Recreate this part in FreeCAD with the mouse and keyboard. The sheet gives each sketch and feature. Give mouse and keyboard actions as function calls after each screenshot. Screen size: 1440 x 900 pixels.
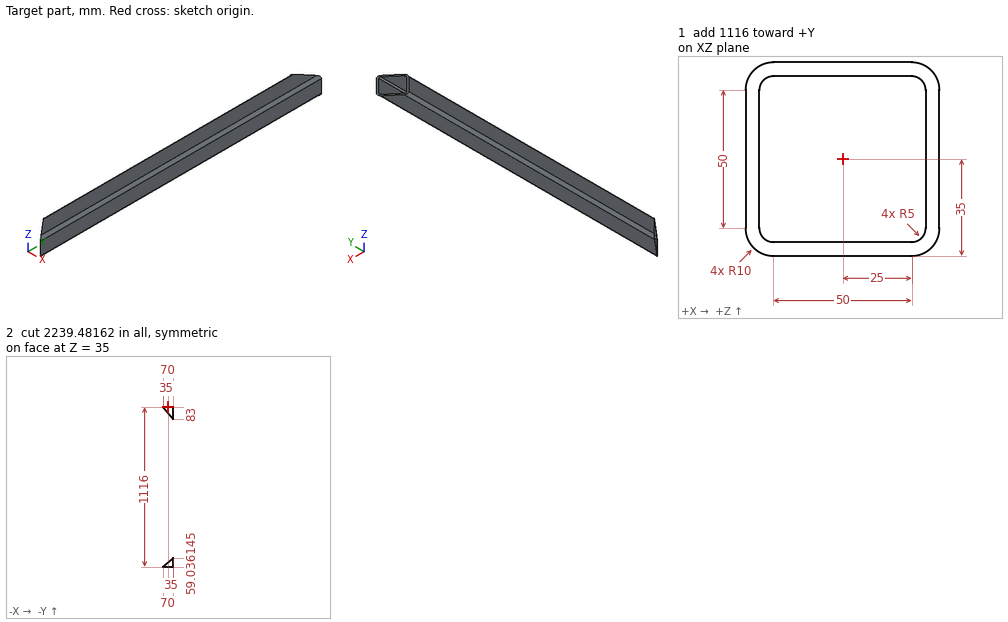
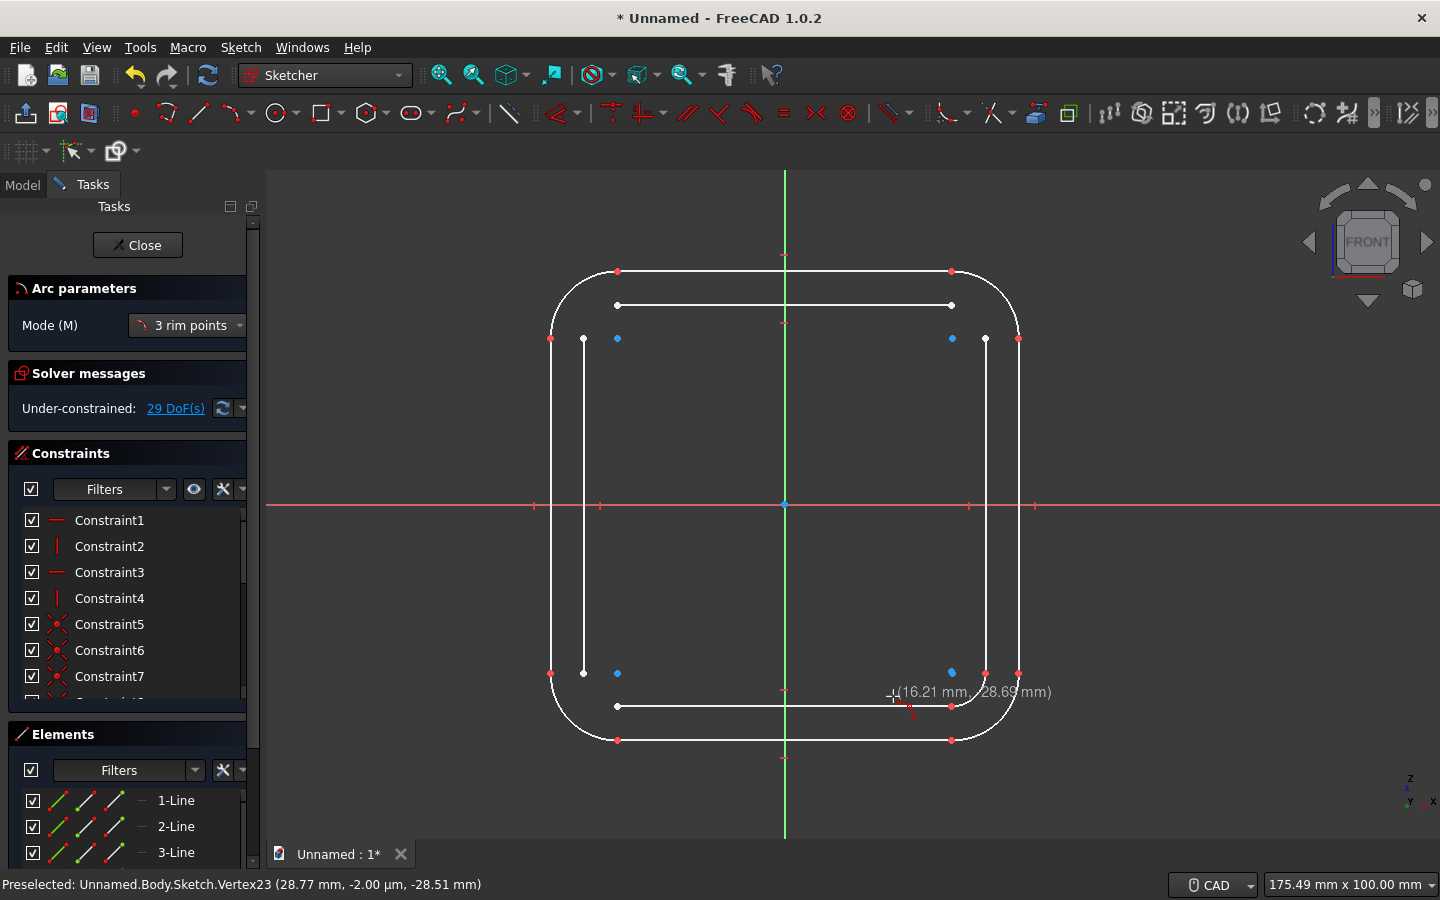
click(986, 338)
click(952, 305)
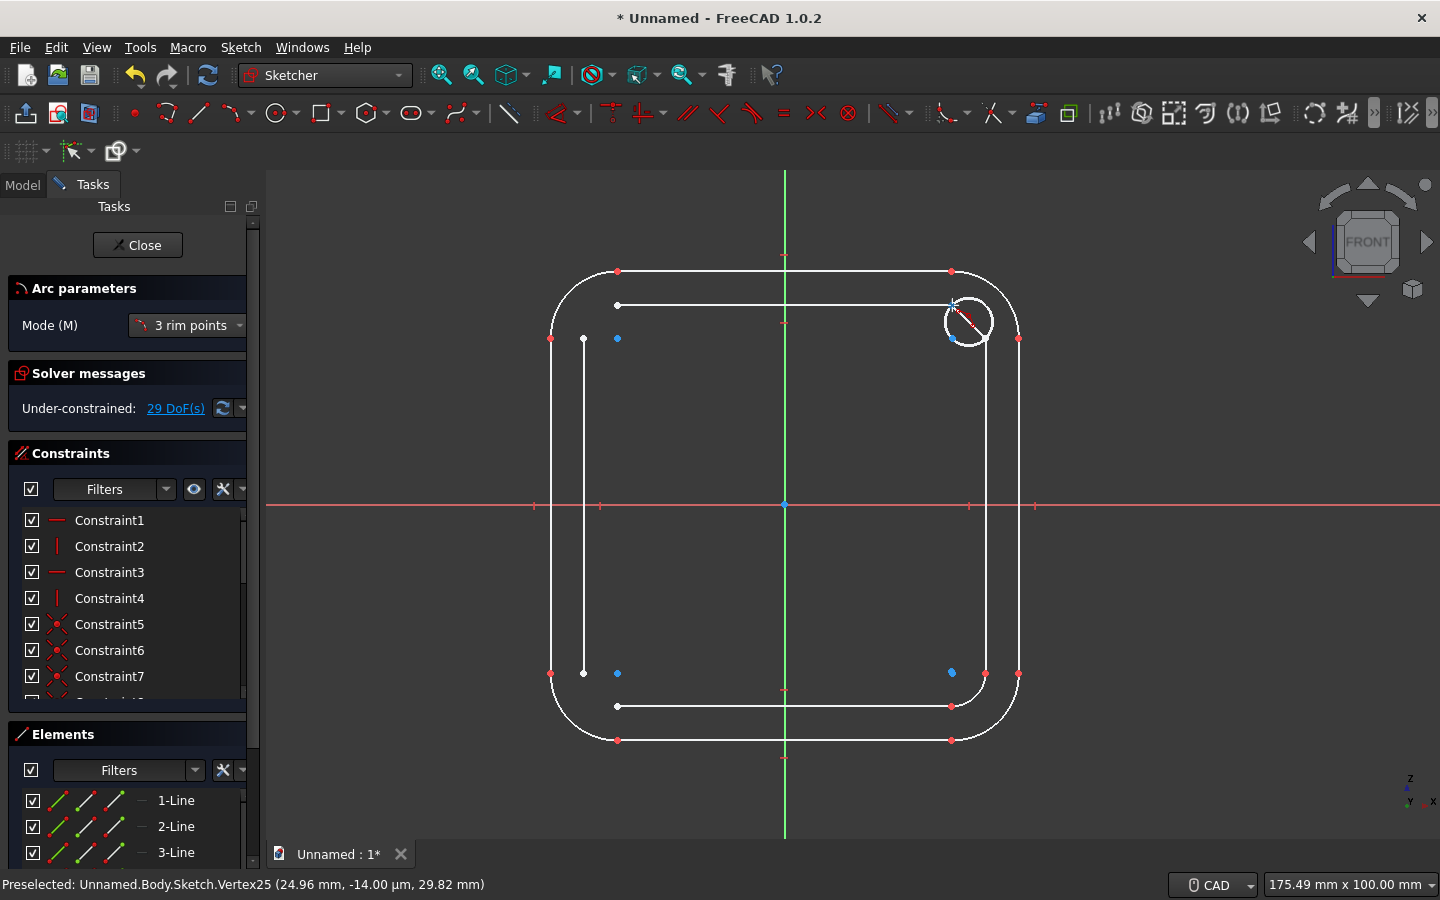
scroll(976, 314, up, 3)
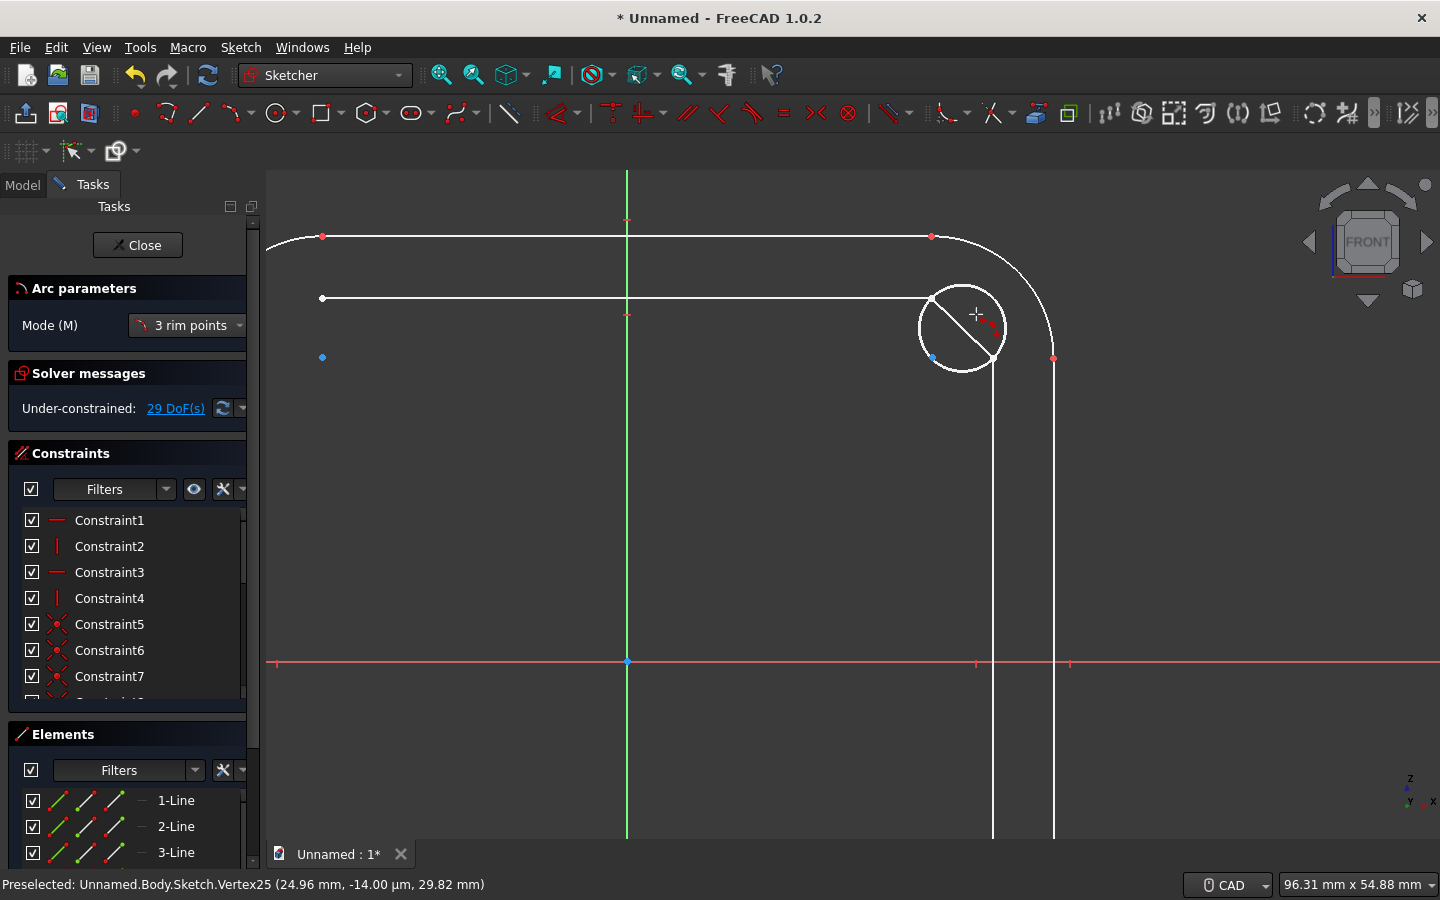
click(975, 314)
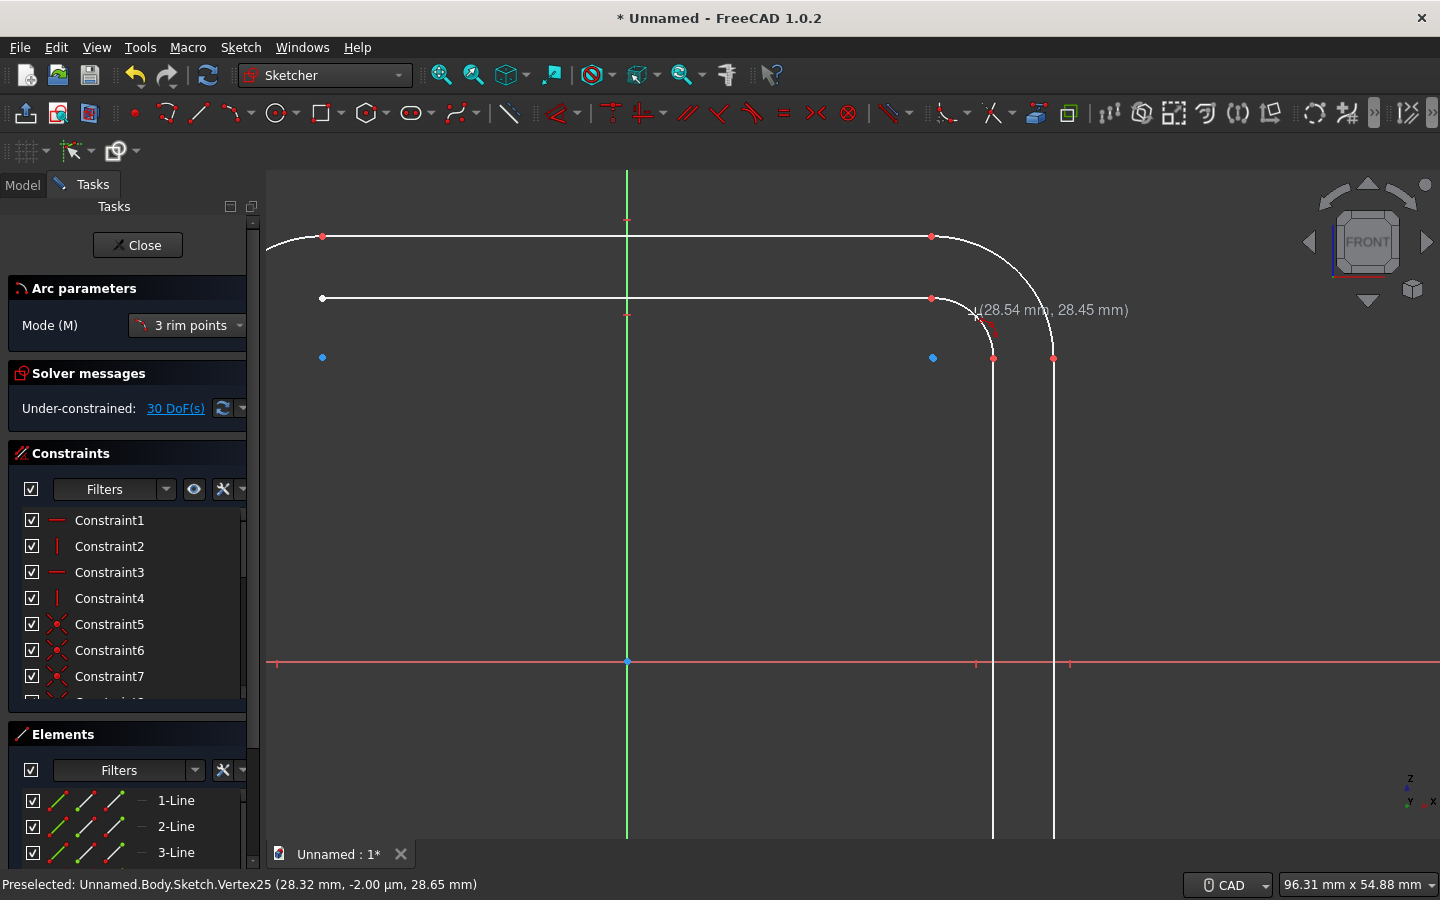
click(323, 298)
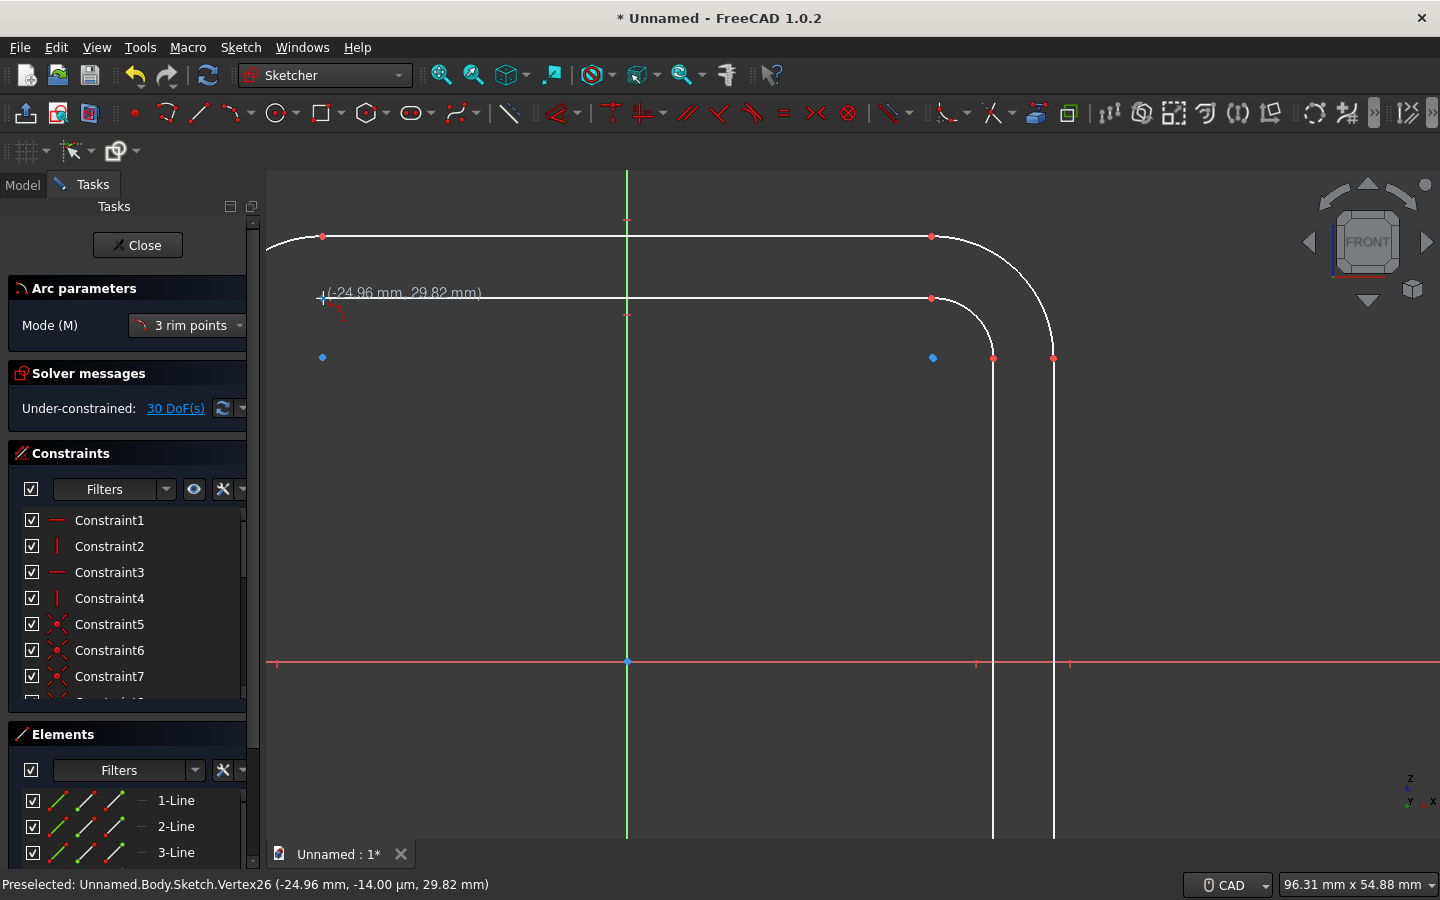
scroll(976, 313, down, 3)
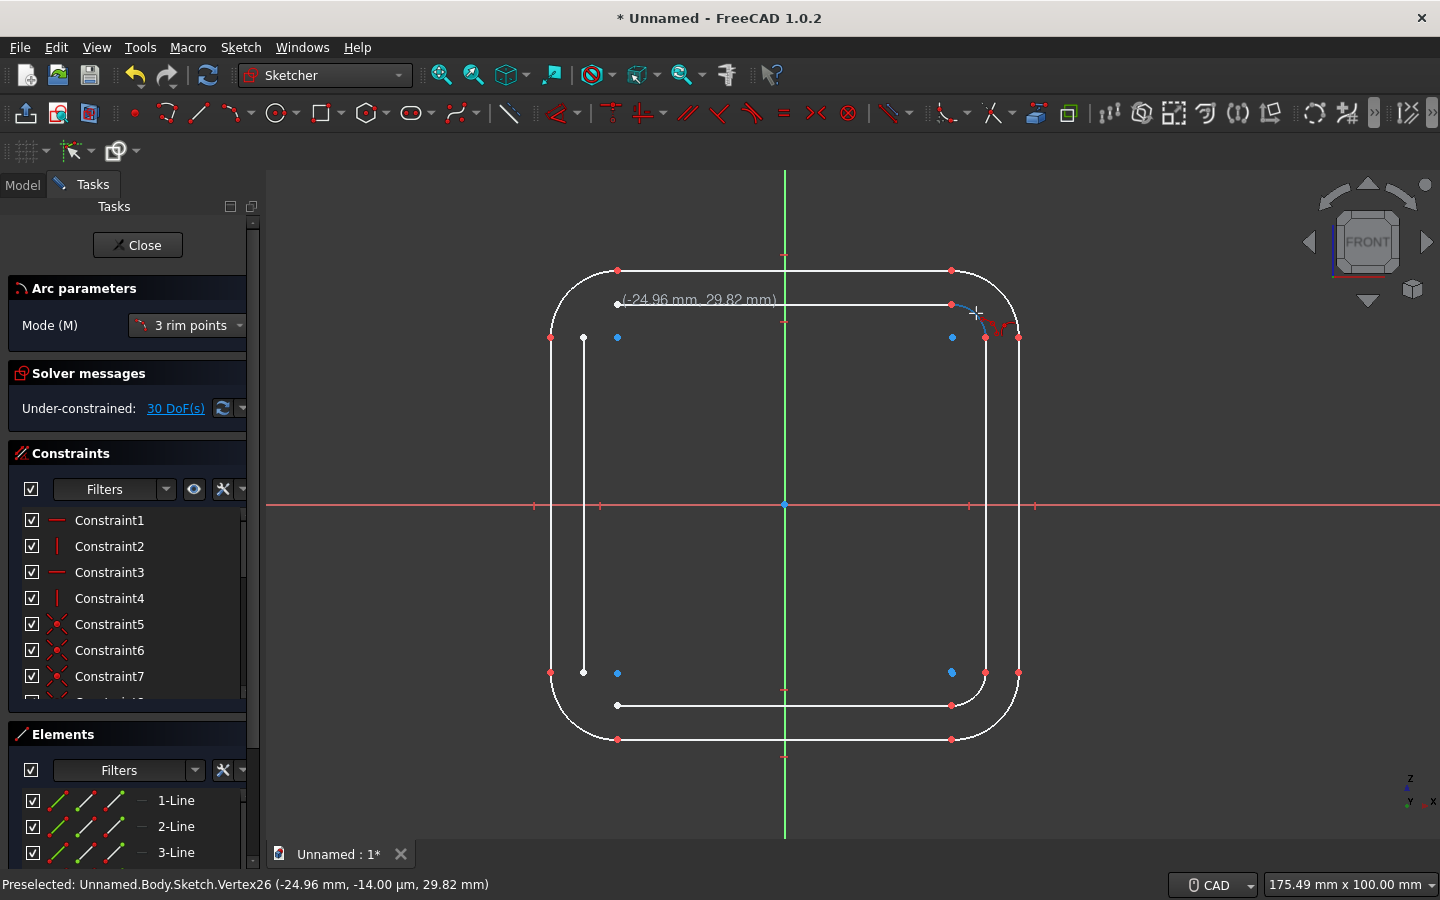
click(584, 338)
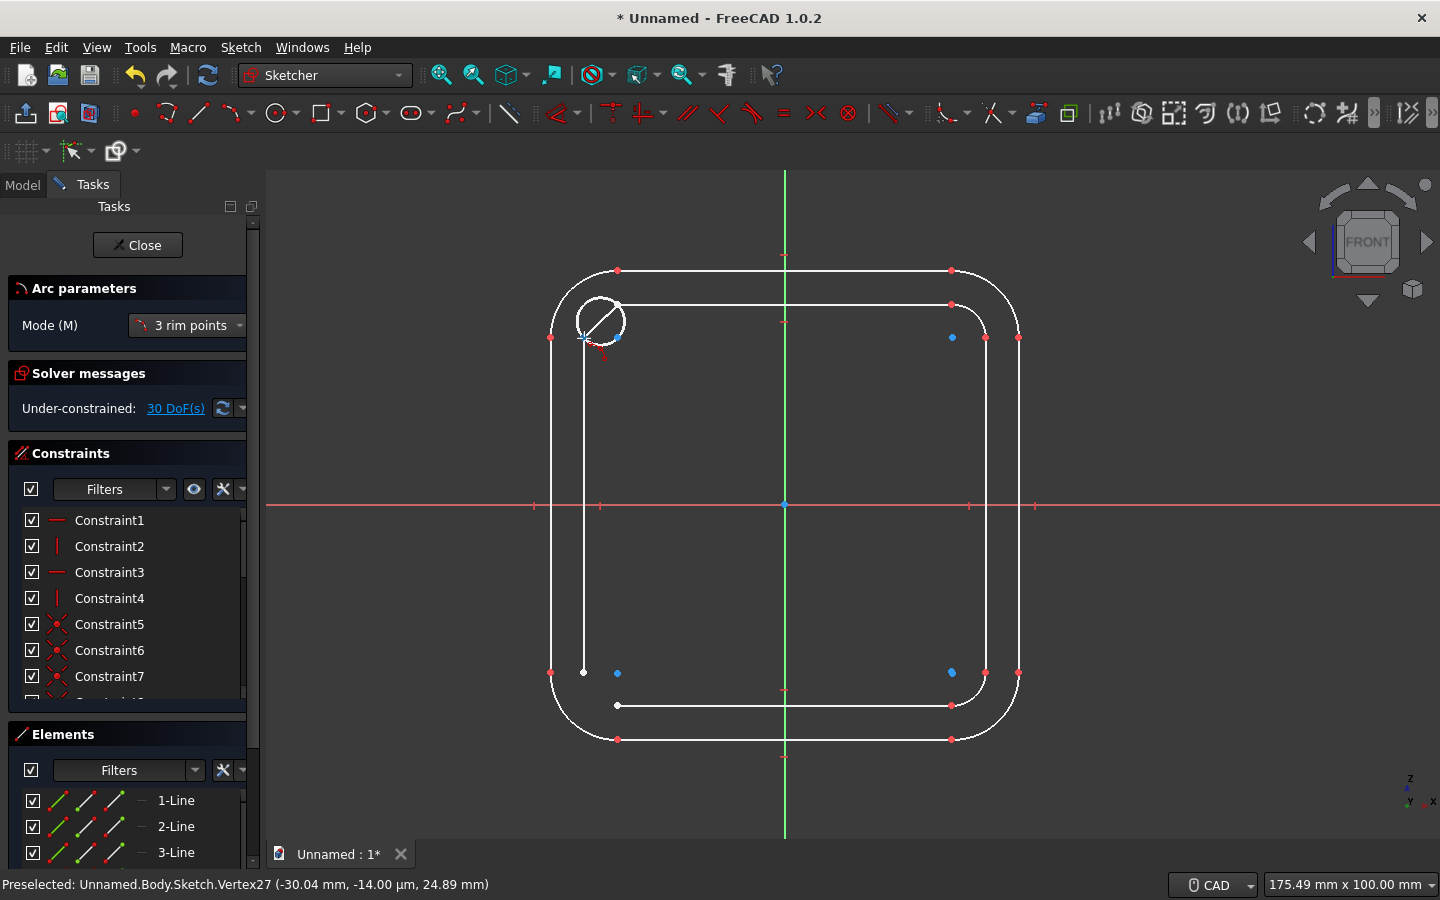
scroll(594, 314, up, 3)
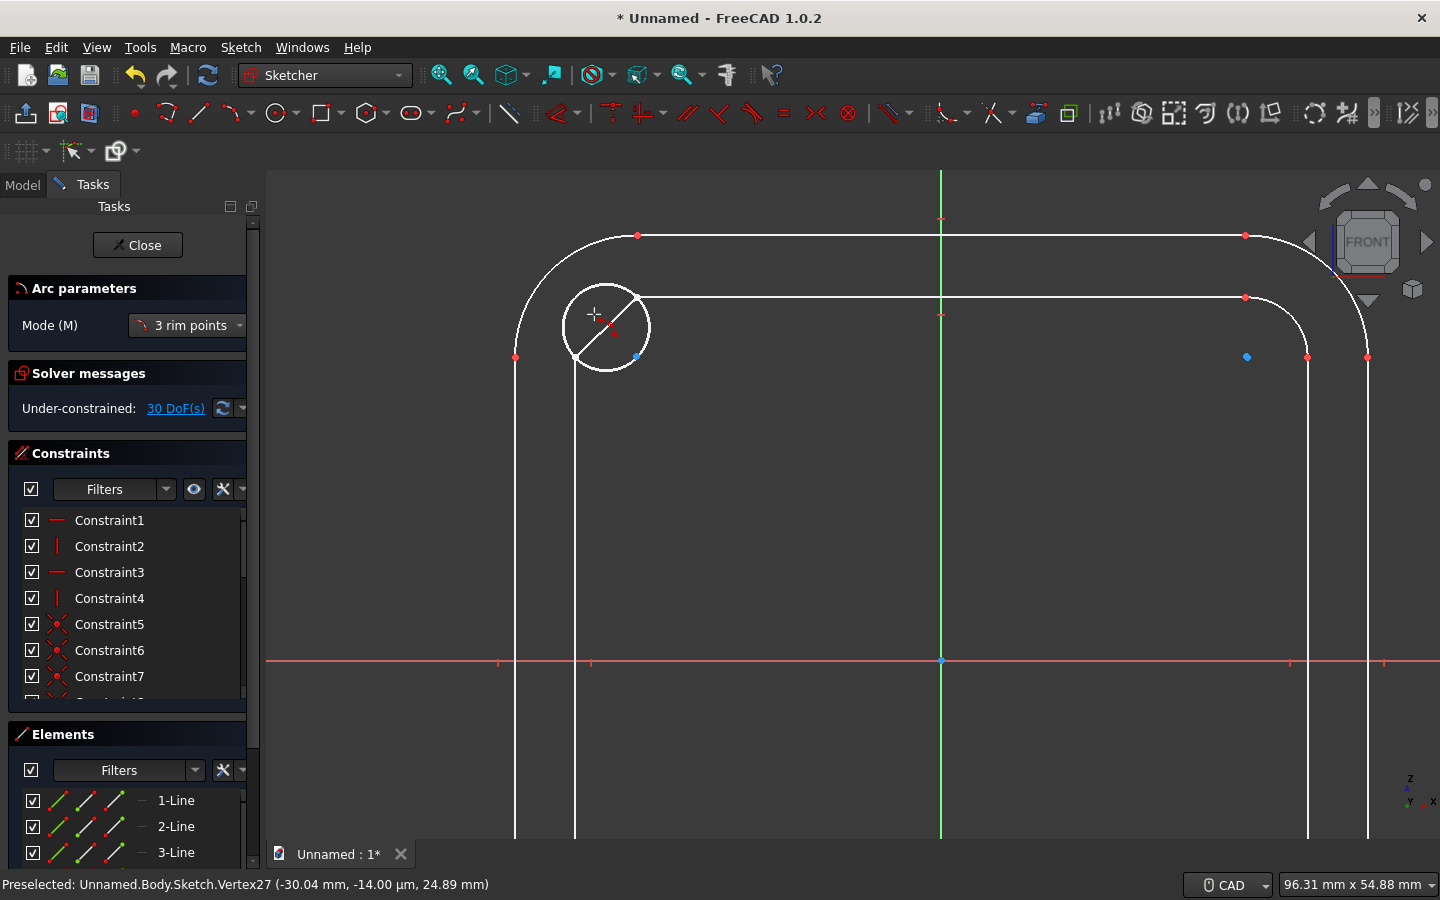
click(594, 313)